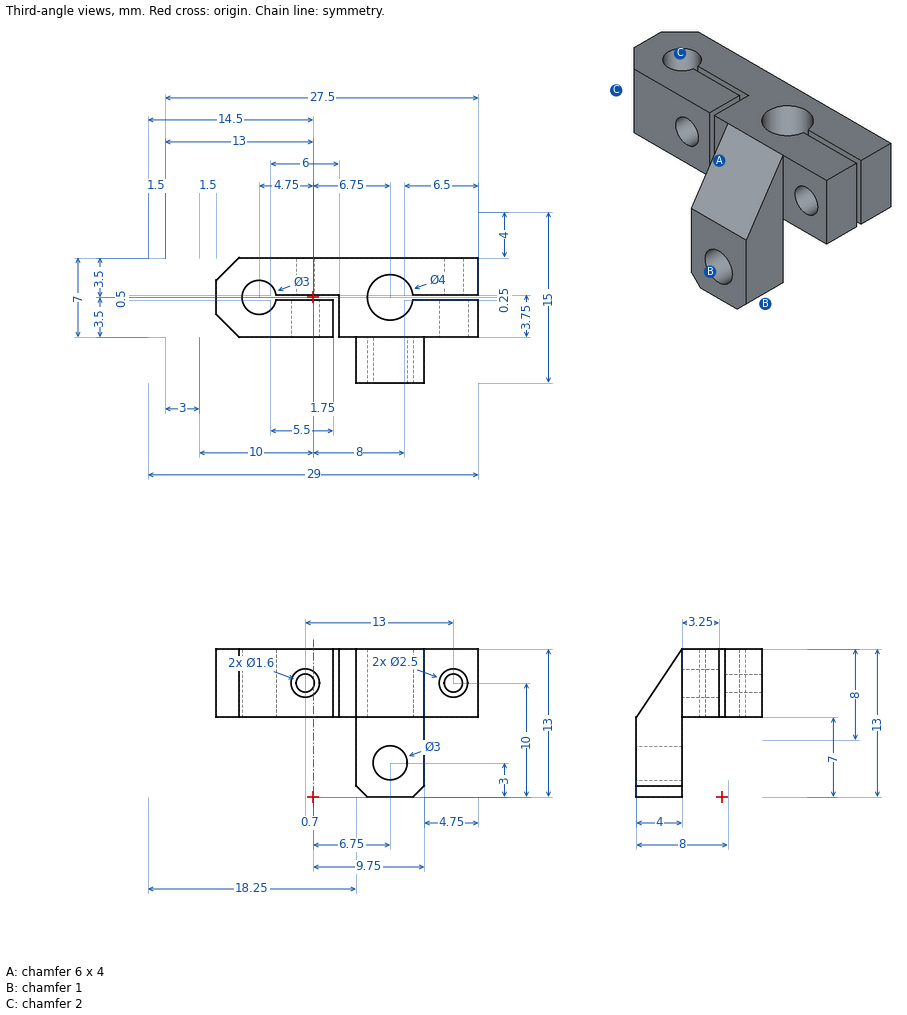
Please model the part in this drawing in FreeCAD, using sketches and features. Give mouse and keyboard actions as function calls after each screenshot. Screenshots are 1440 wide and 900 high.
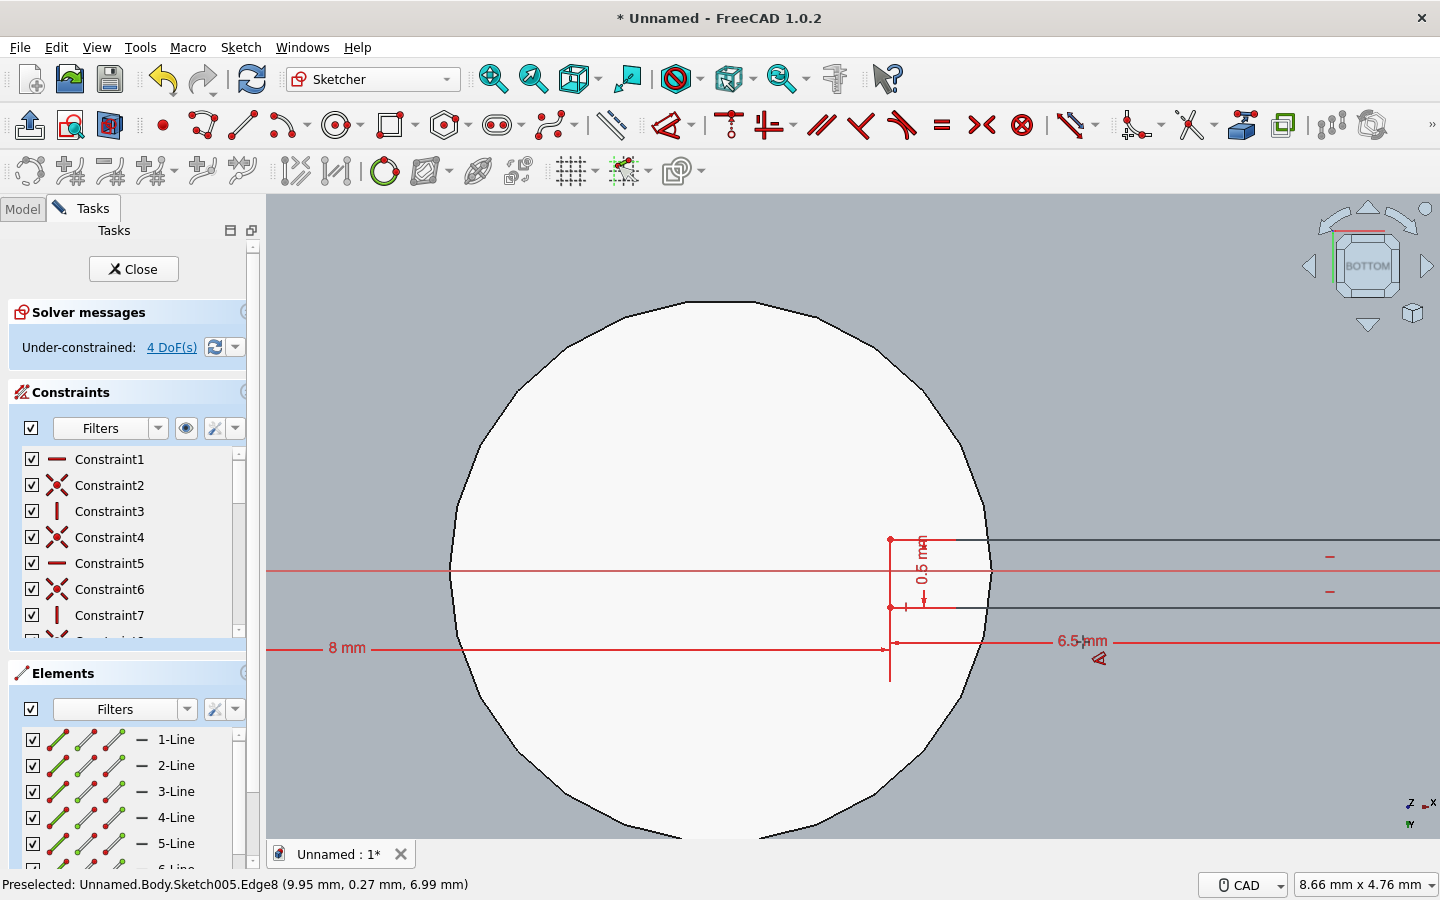
scroll(892, 588, down, 6)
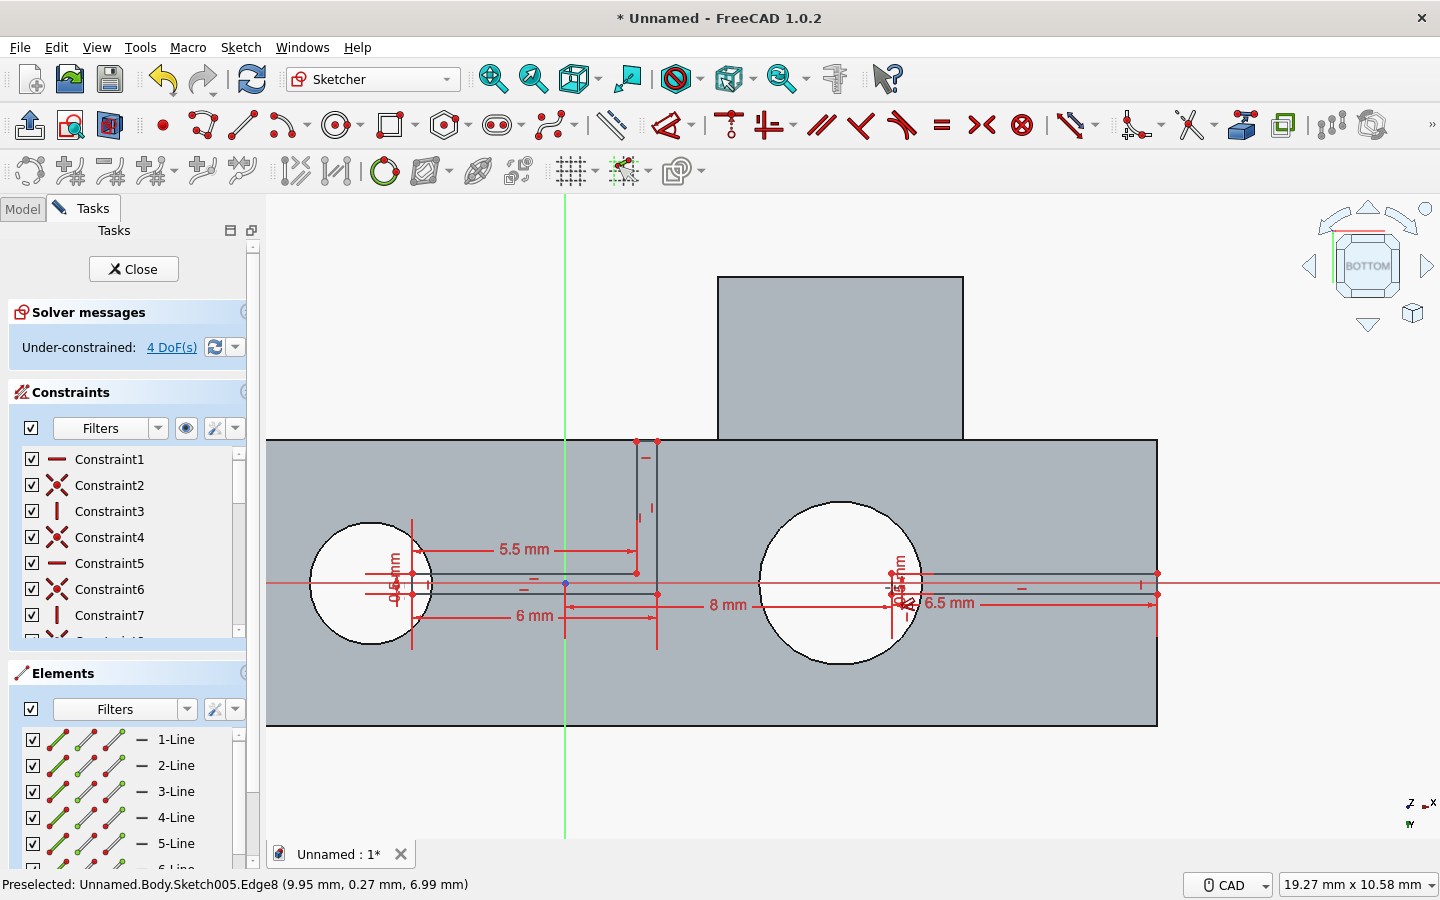
click(657, 548)
click(623, 518)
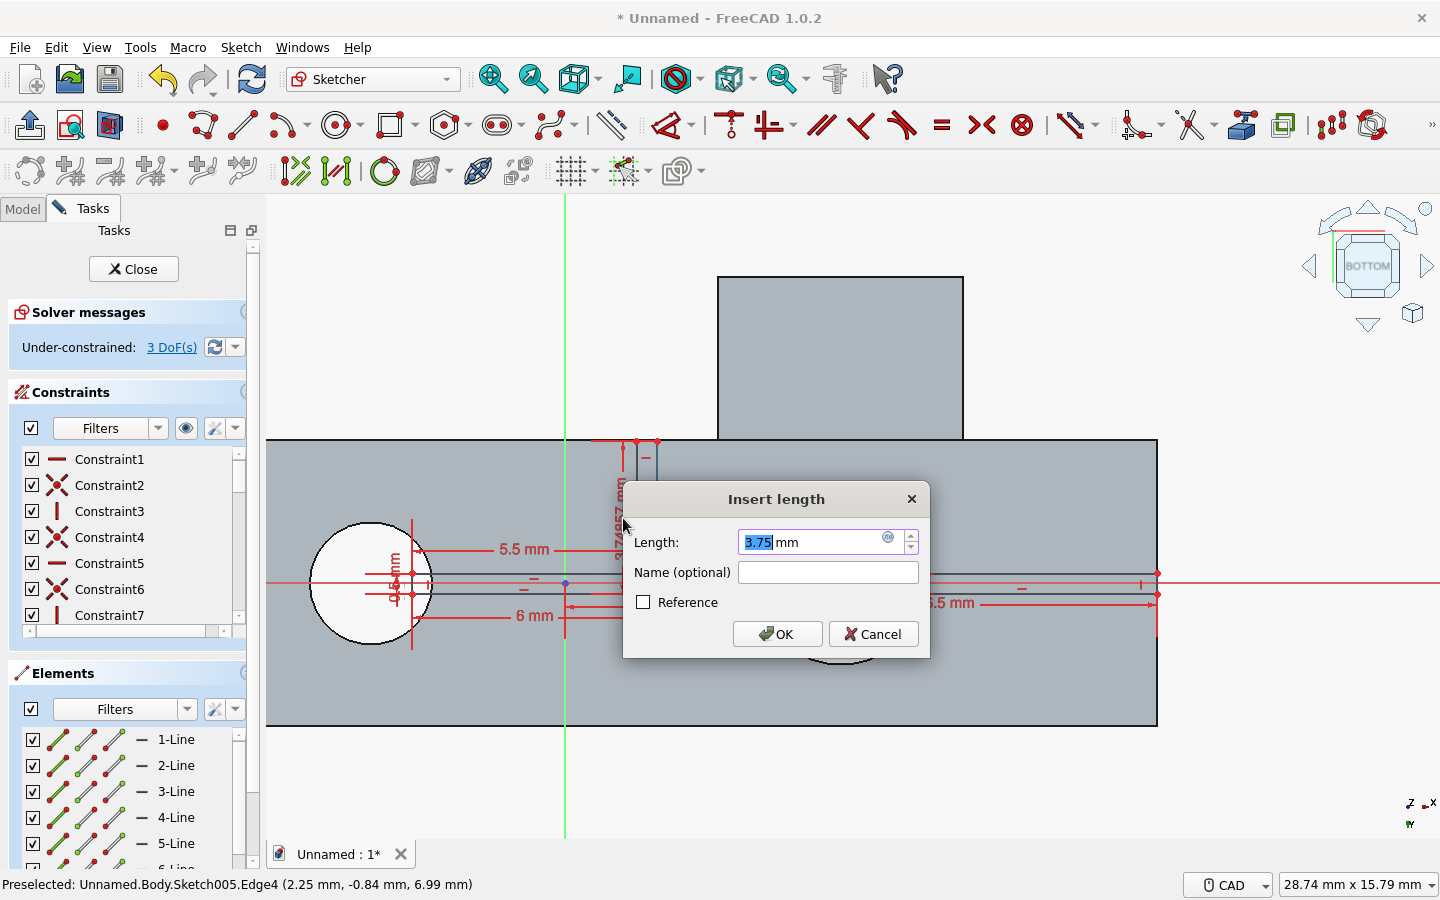
text(3.75)
key(Return)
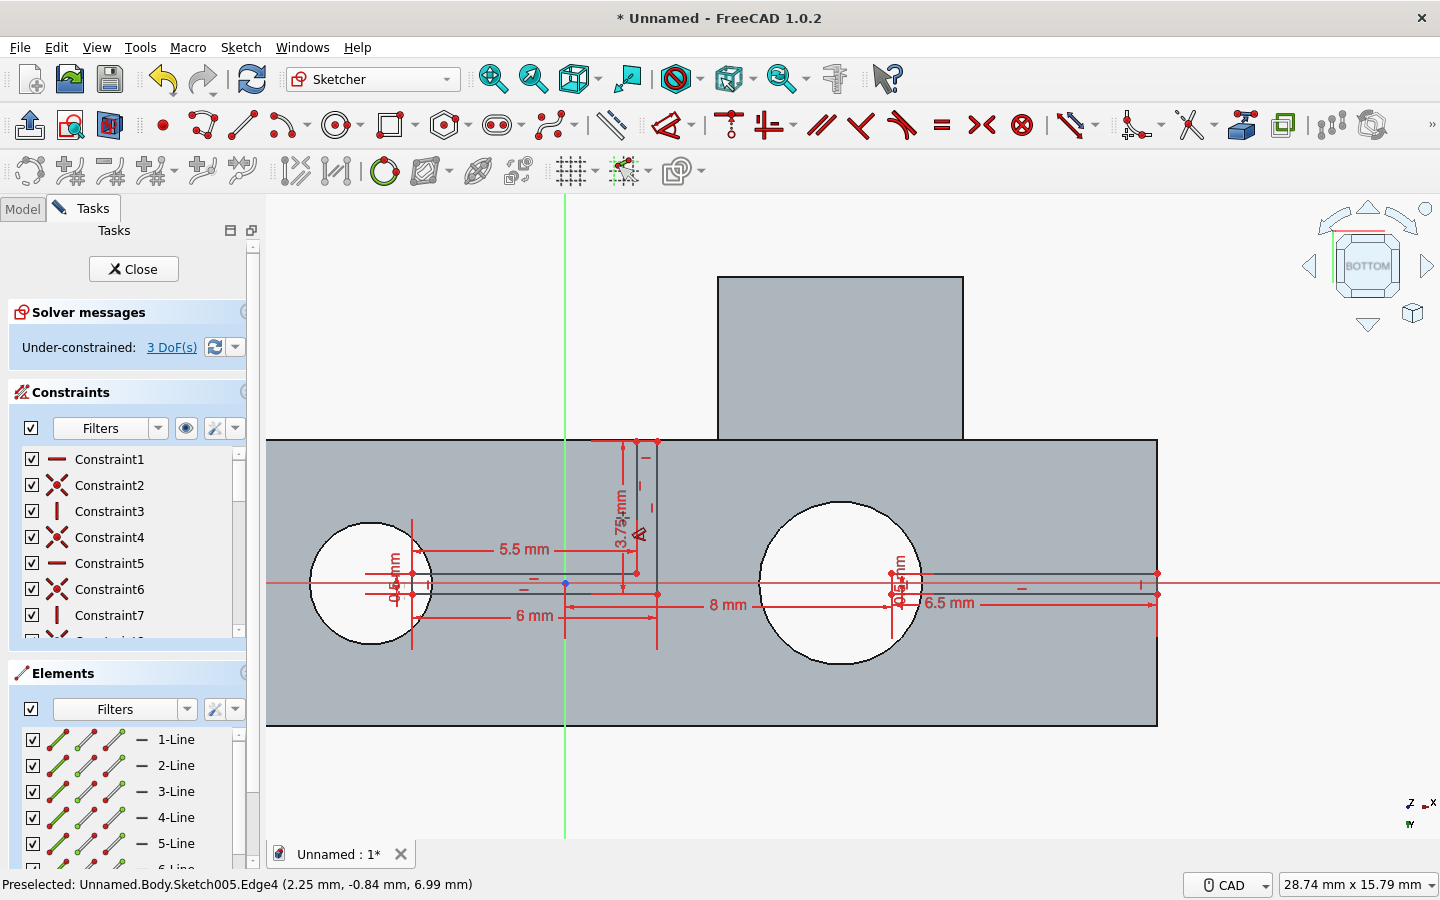
click(657, 441)
click(531, 512)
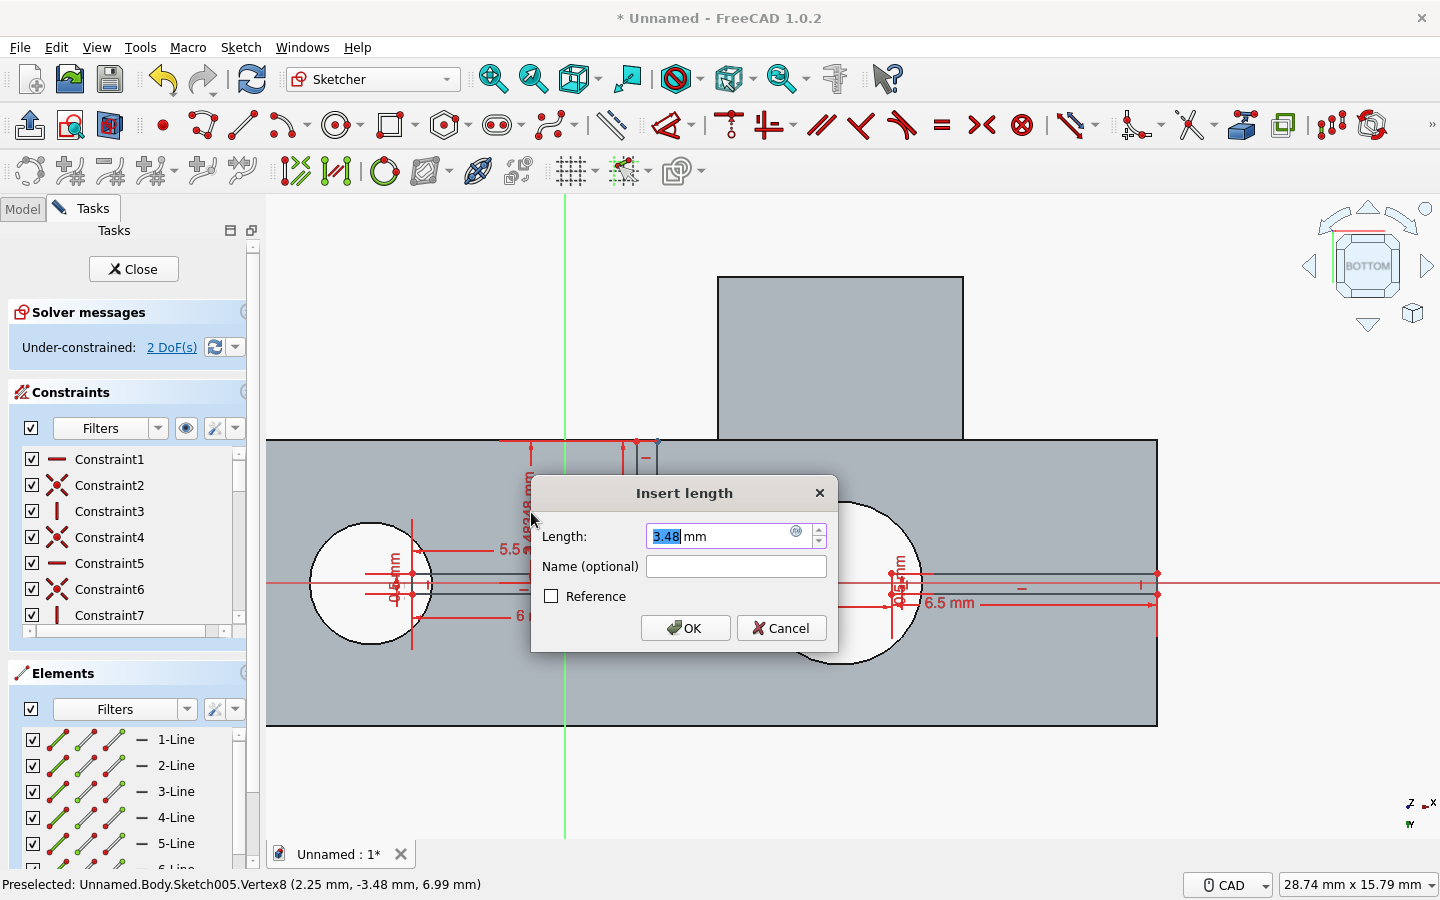
text(3.5)
key(Return)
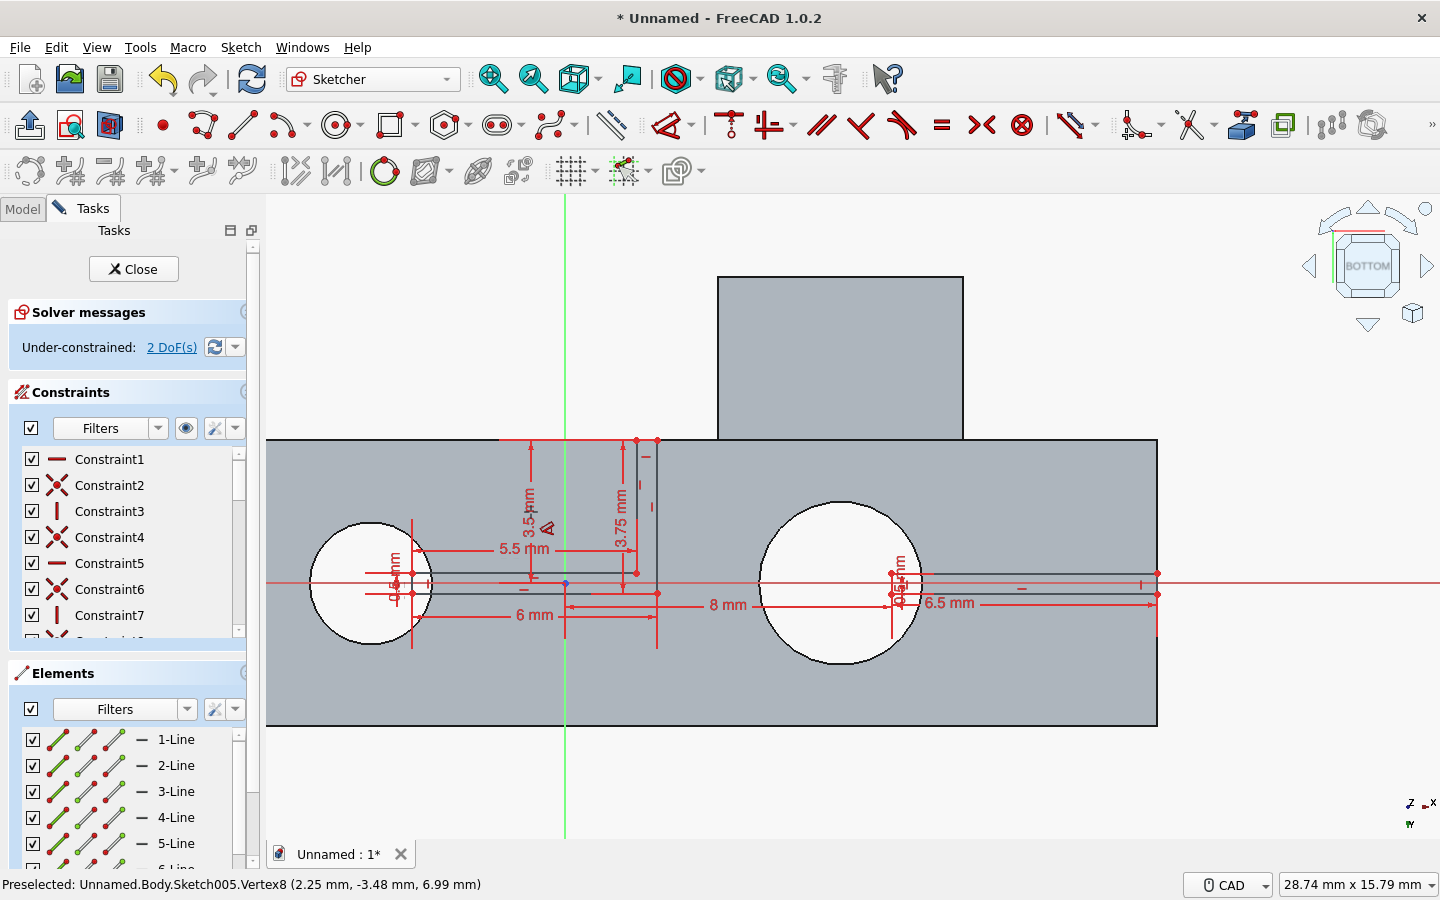
click(637, 573)
click(617, 617)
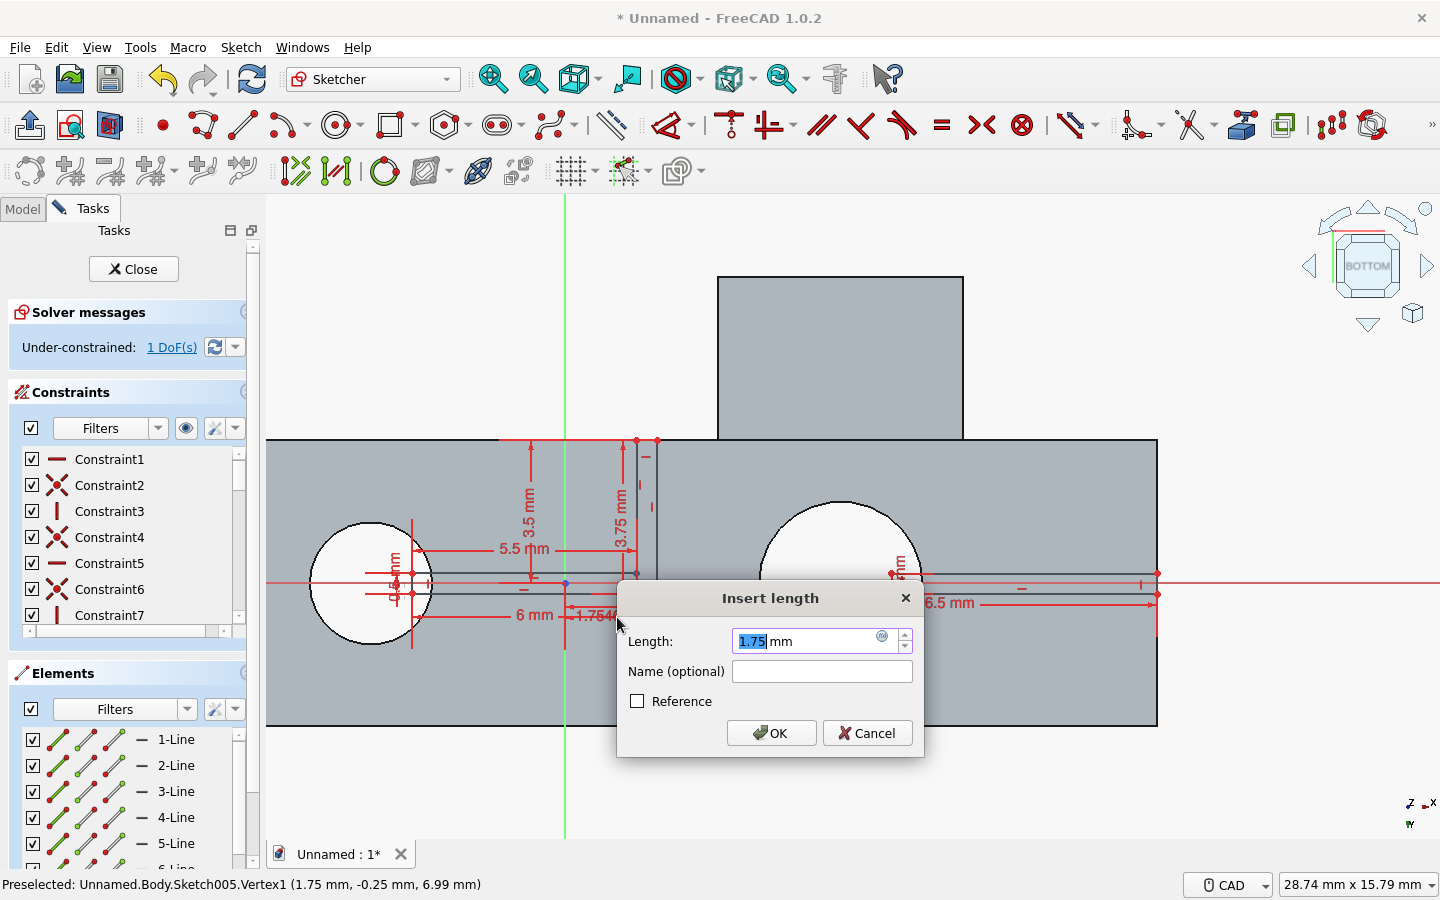
text(1.75)
key(Return)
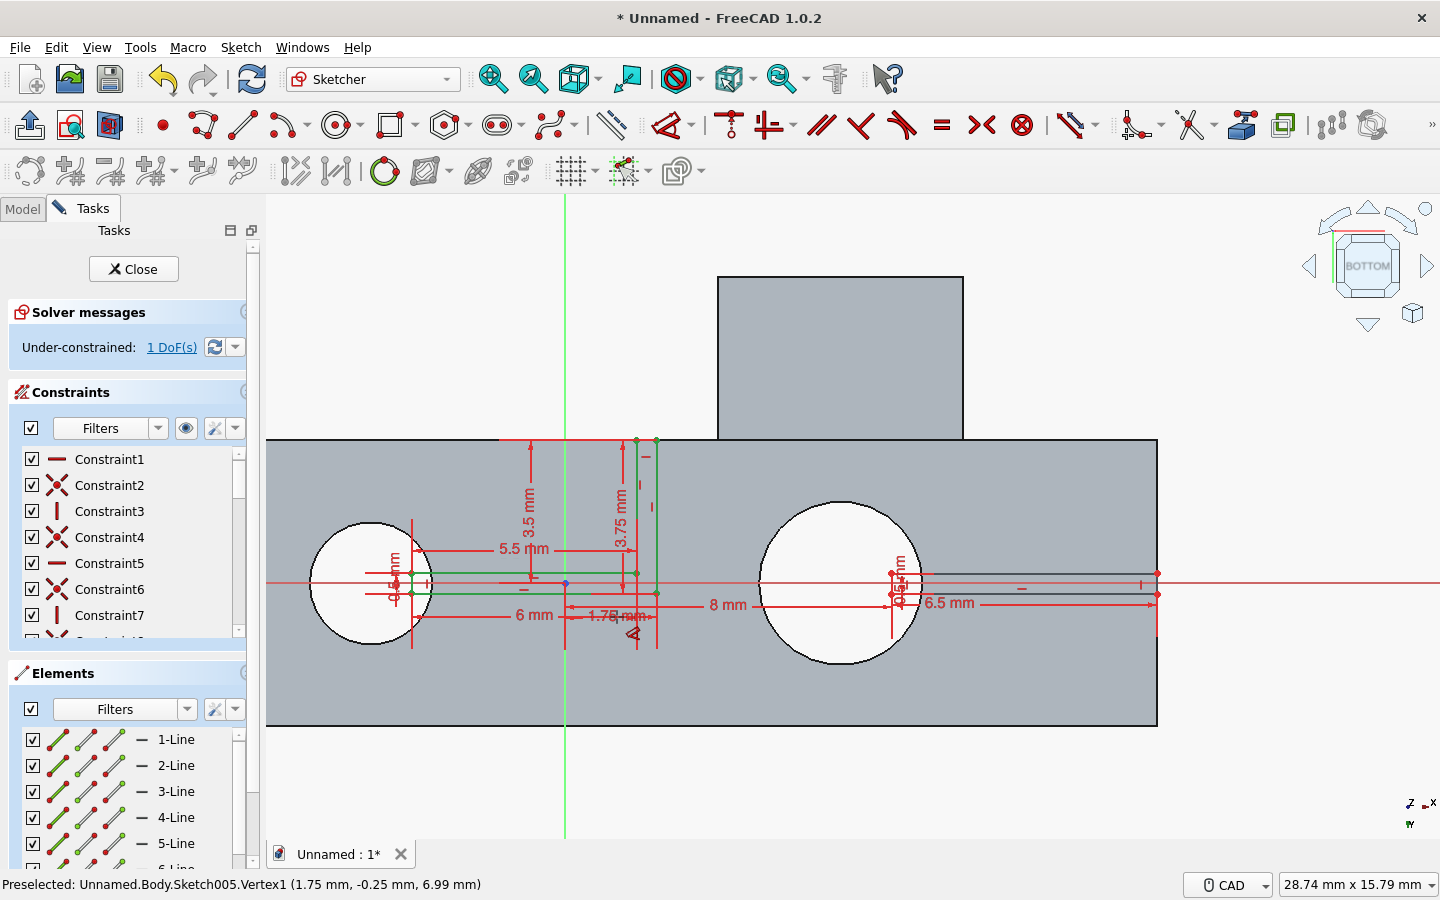
scroll(892, 574, up, 7)